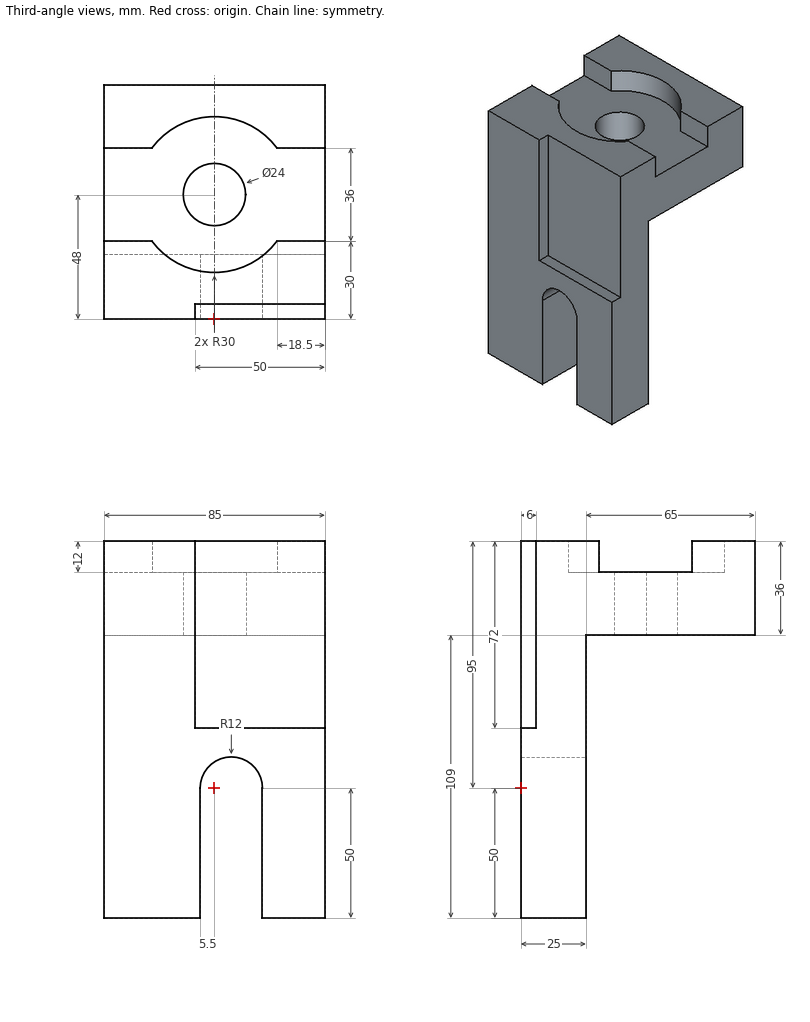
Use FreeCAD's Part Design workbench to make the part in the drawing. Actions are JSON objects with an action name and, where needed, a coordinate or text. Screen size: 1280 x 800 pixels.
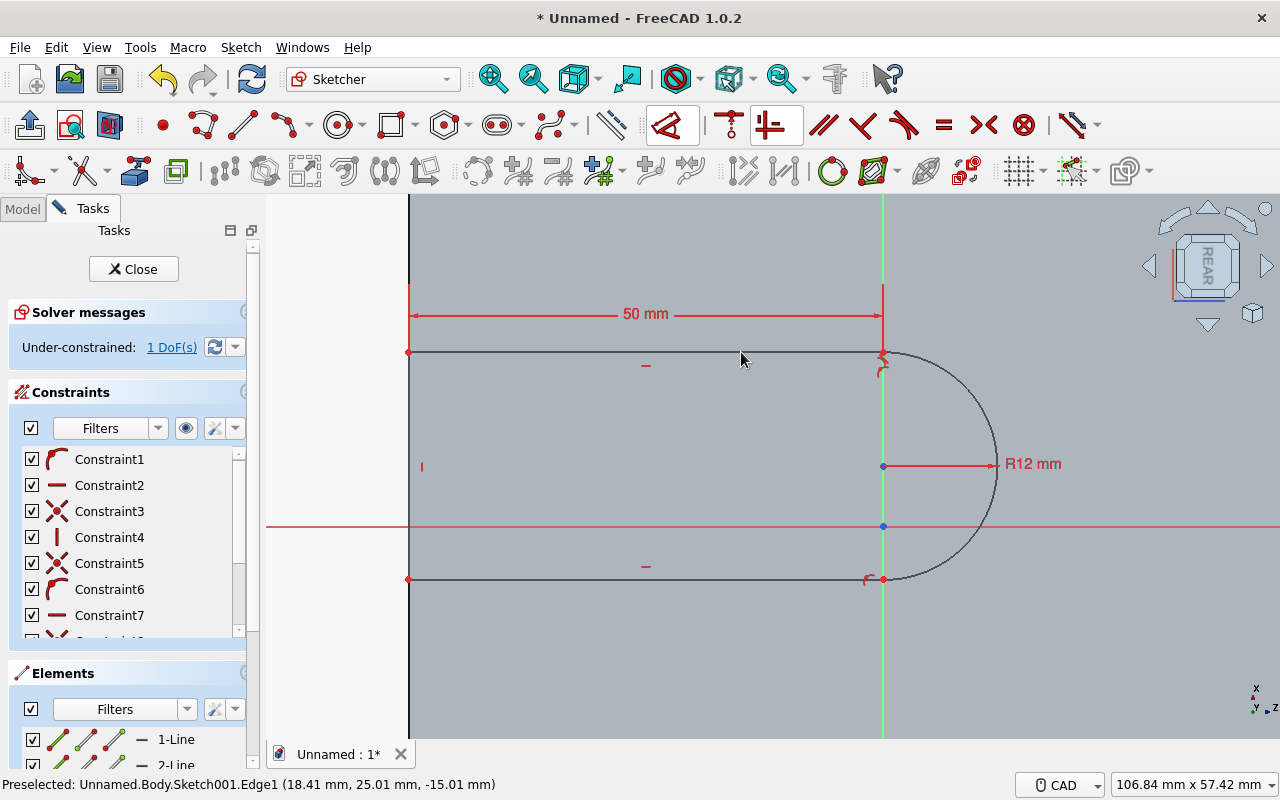
{"action": "left_click", "coordinate": [409, 580]}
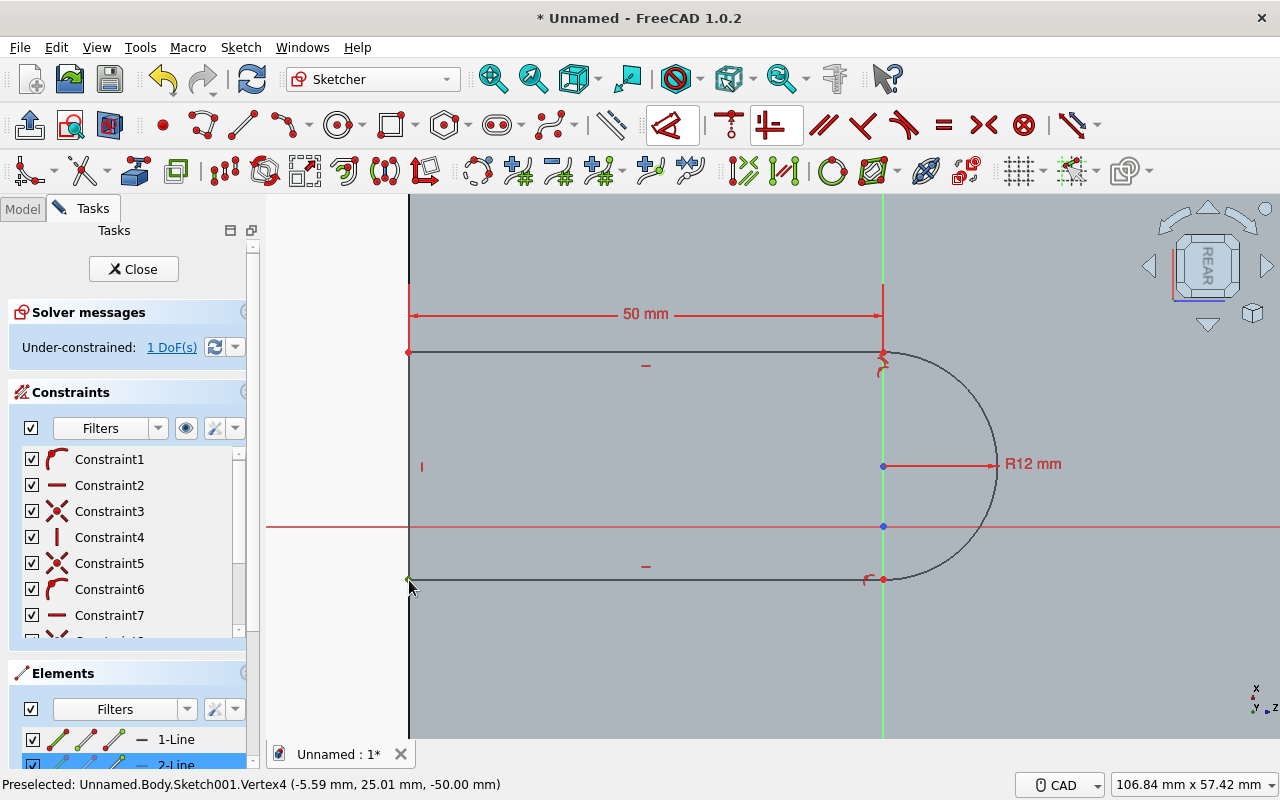
{"action": "left_click", "coordinate": [694, 126]}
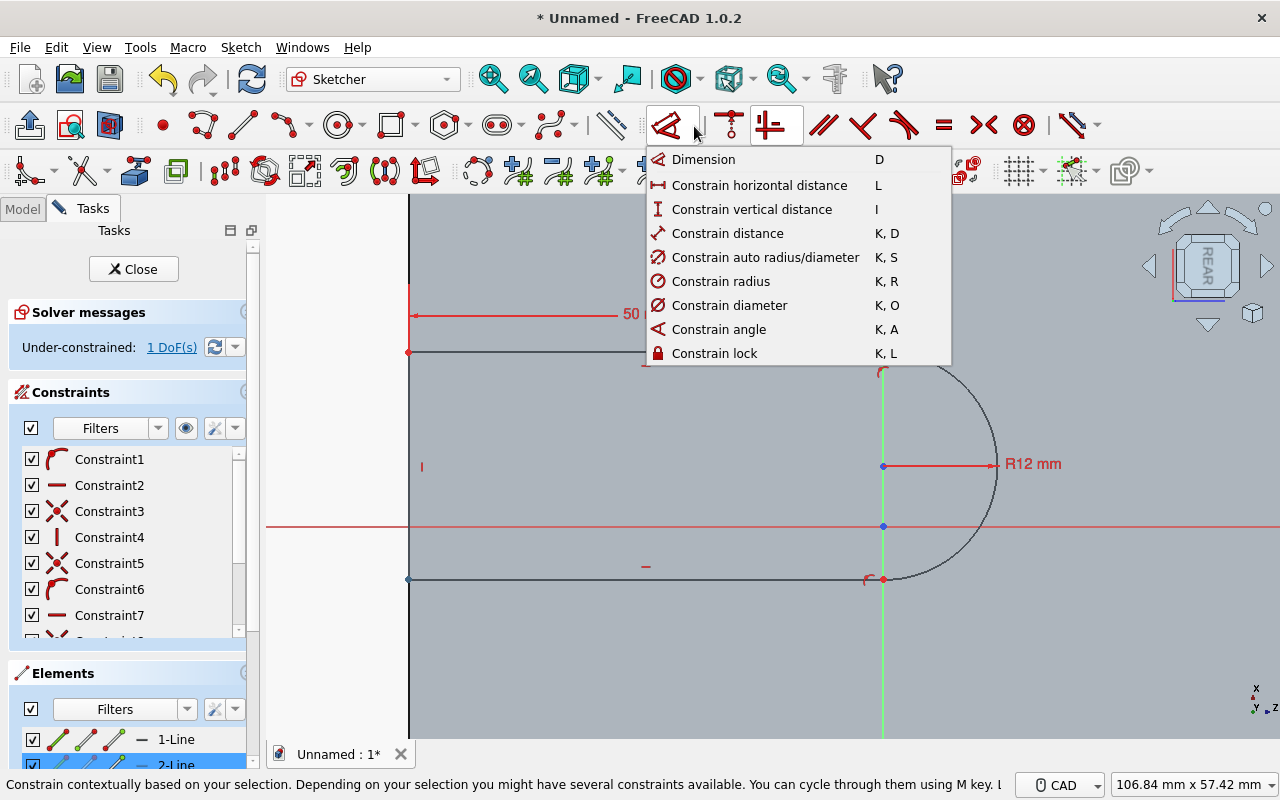
{"action": "left_click", "coordinate": [799, 209]}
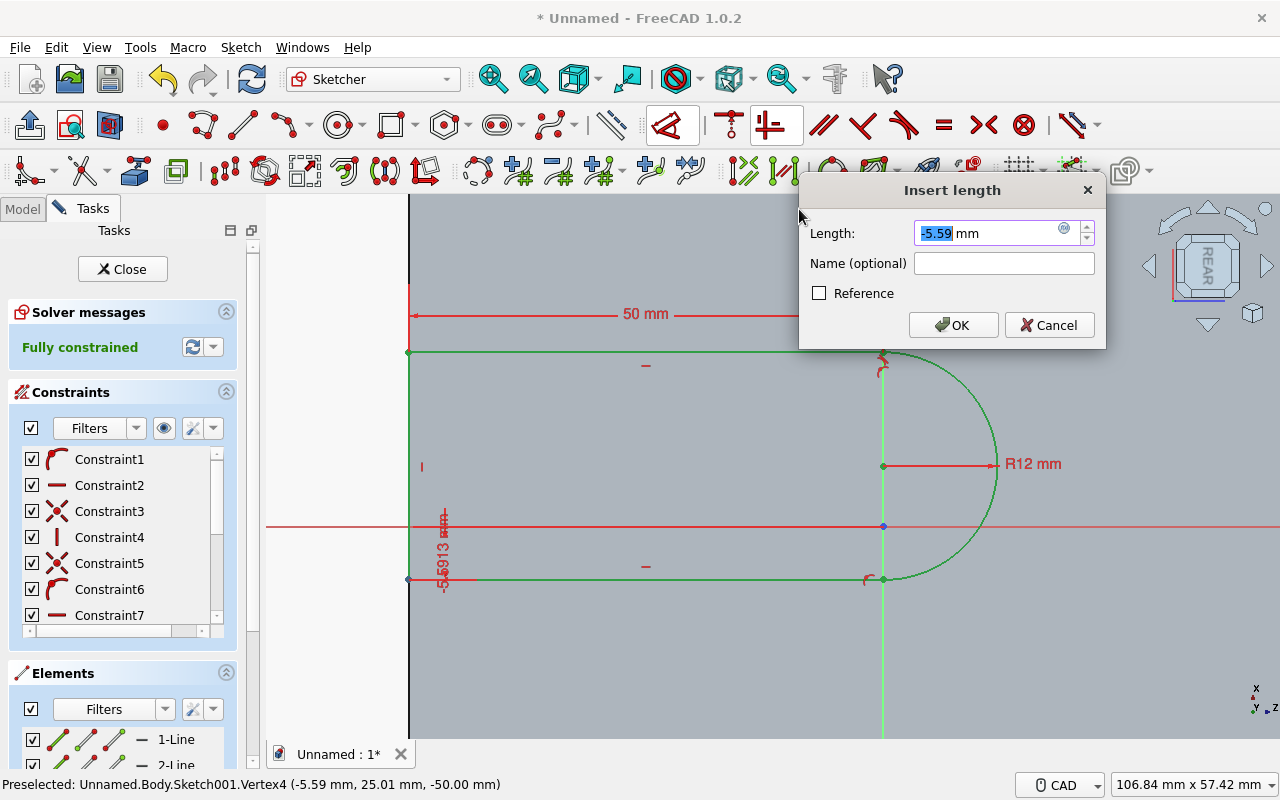
{"action": "type", "text": "-5.5"}
{"action": "key", "text": "Return"}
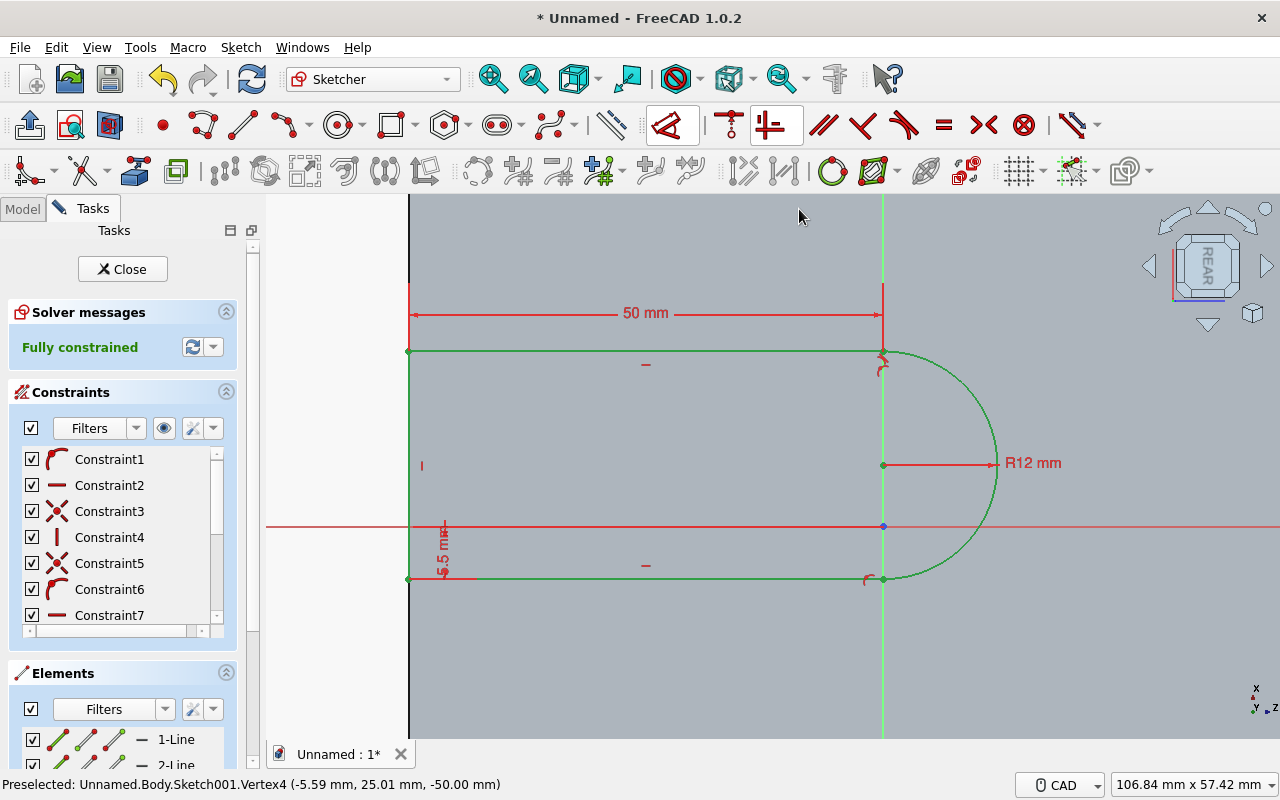
{"action": "left_click", "coordinate": [123, 269]}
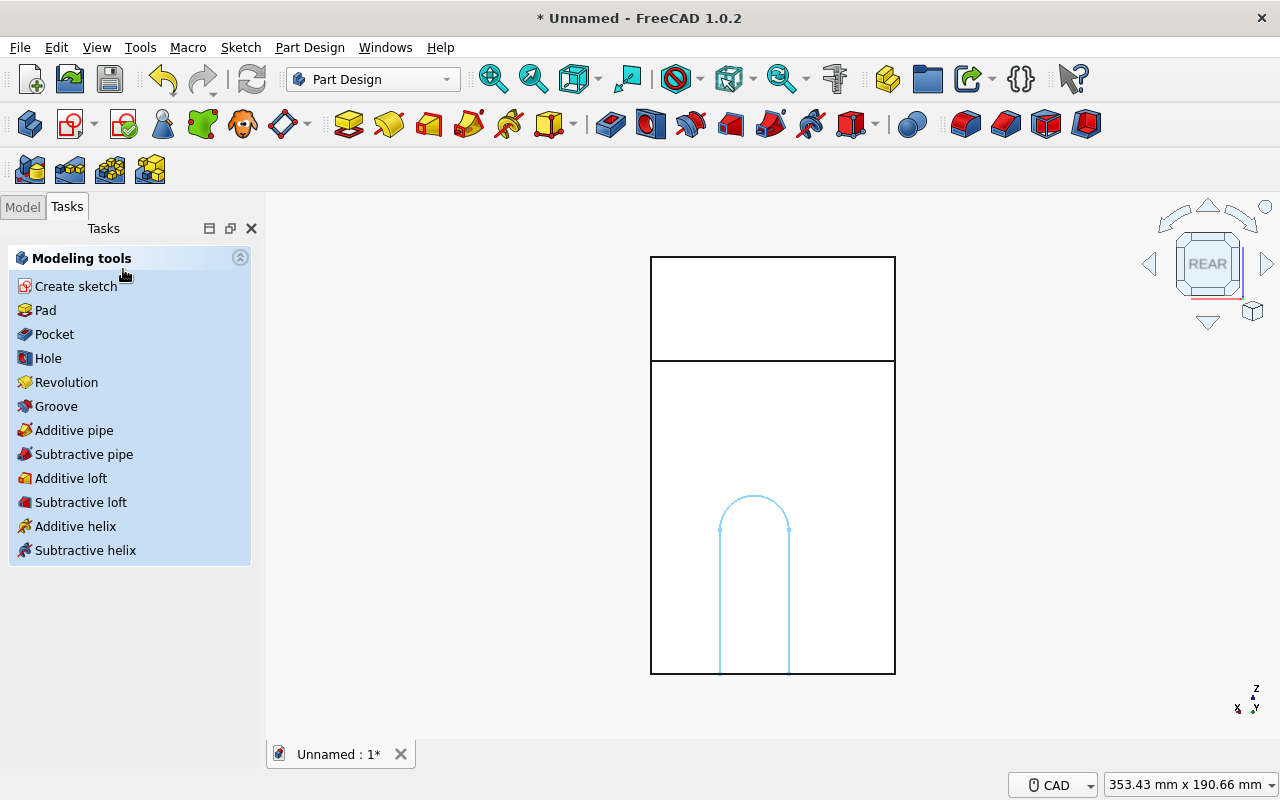
{"action": "left_click", "coordinate": [612, 124]}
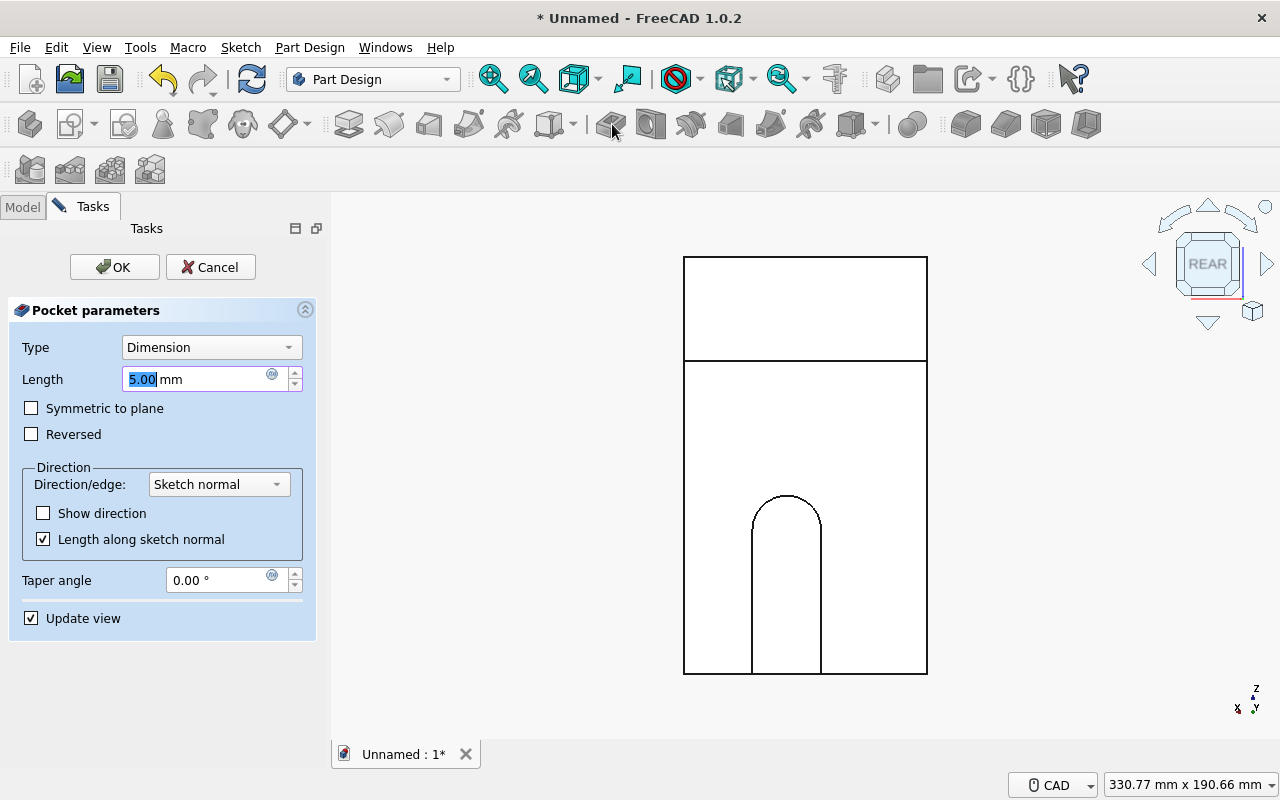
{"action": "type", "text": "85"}
{"action": "key", "text": "Tab"}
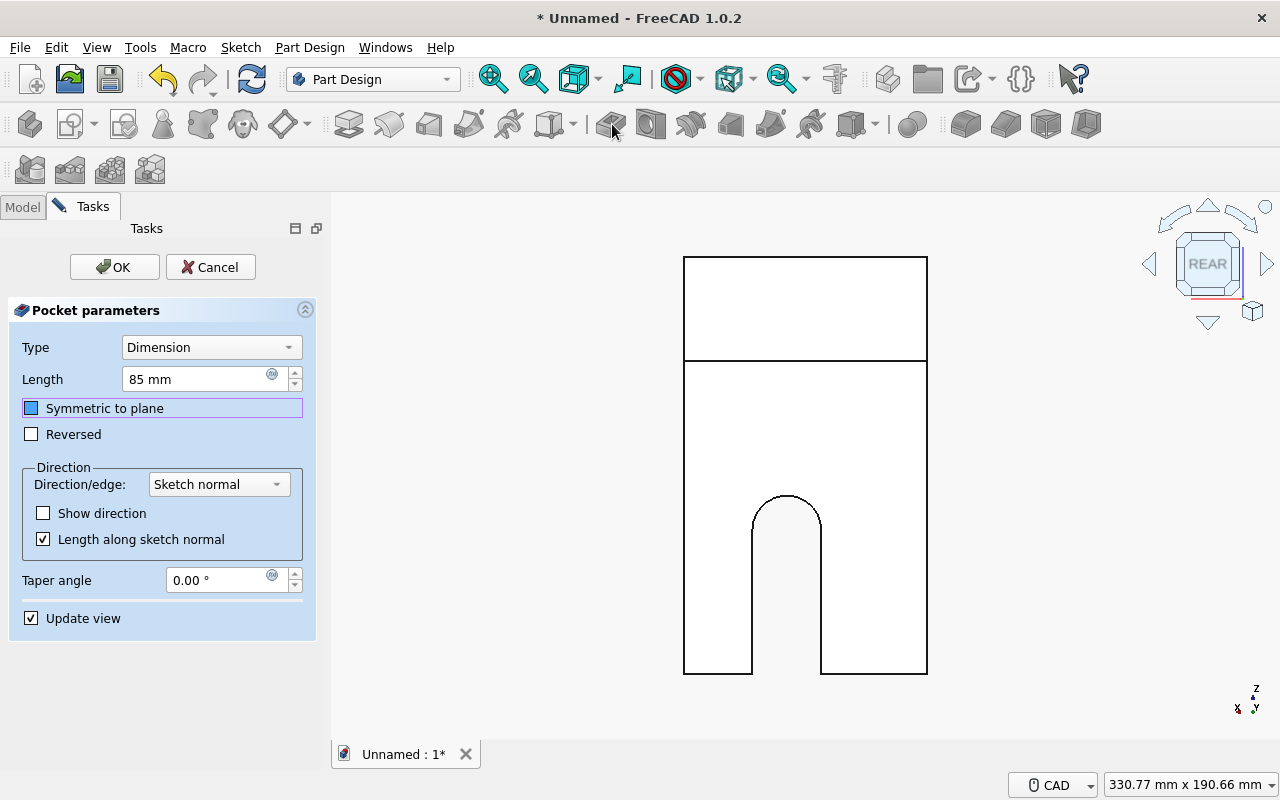
{"action": "left_click", "coordinate": [115, 267]}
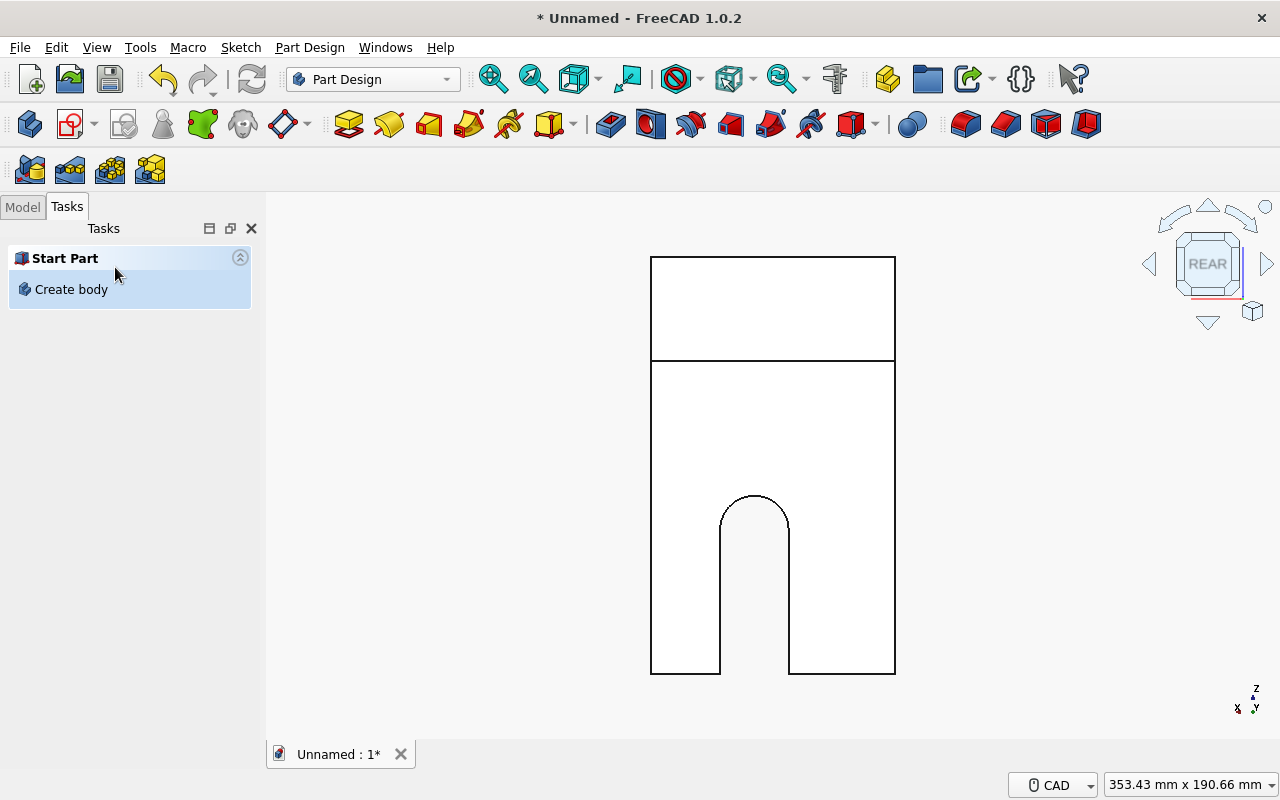
{"action": "key", "text": "0"}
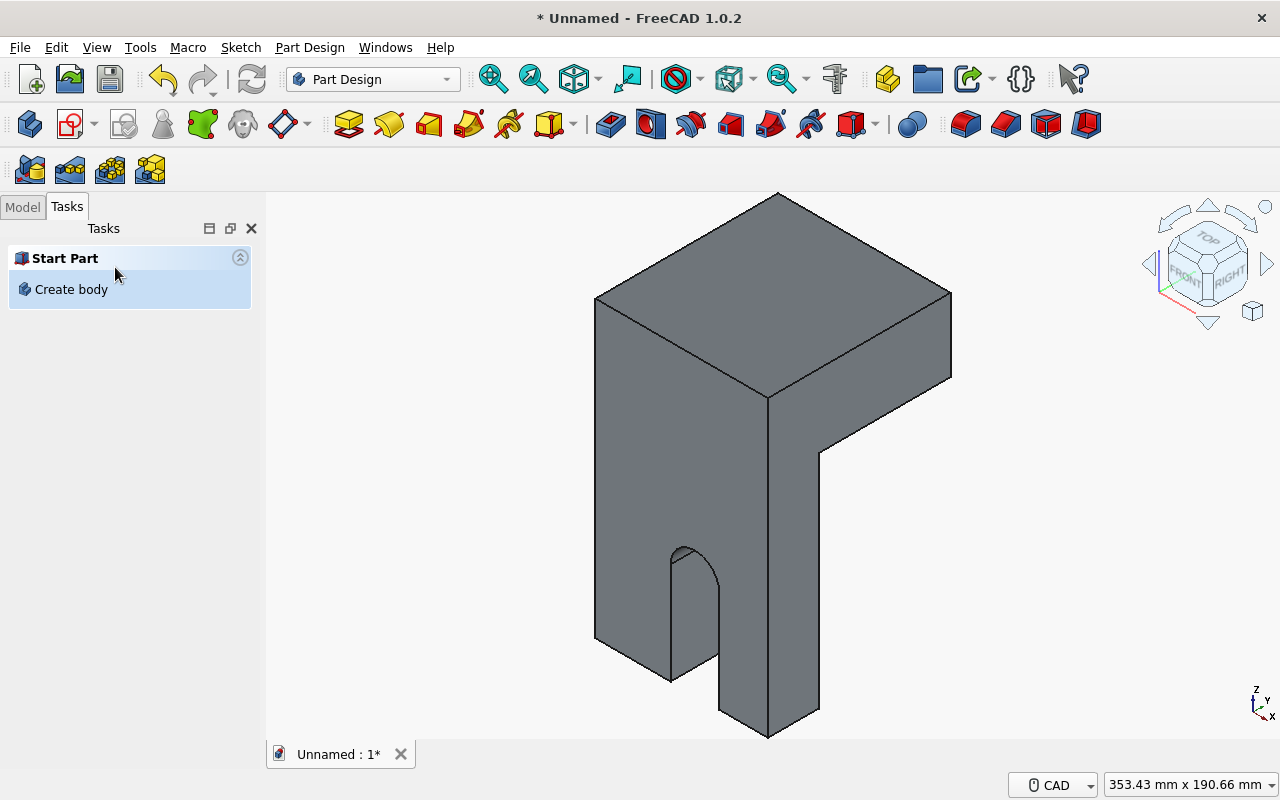
{"action": "left_click", "coordinate": [885, 354]}